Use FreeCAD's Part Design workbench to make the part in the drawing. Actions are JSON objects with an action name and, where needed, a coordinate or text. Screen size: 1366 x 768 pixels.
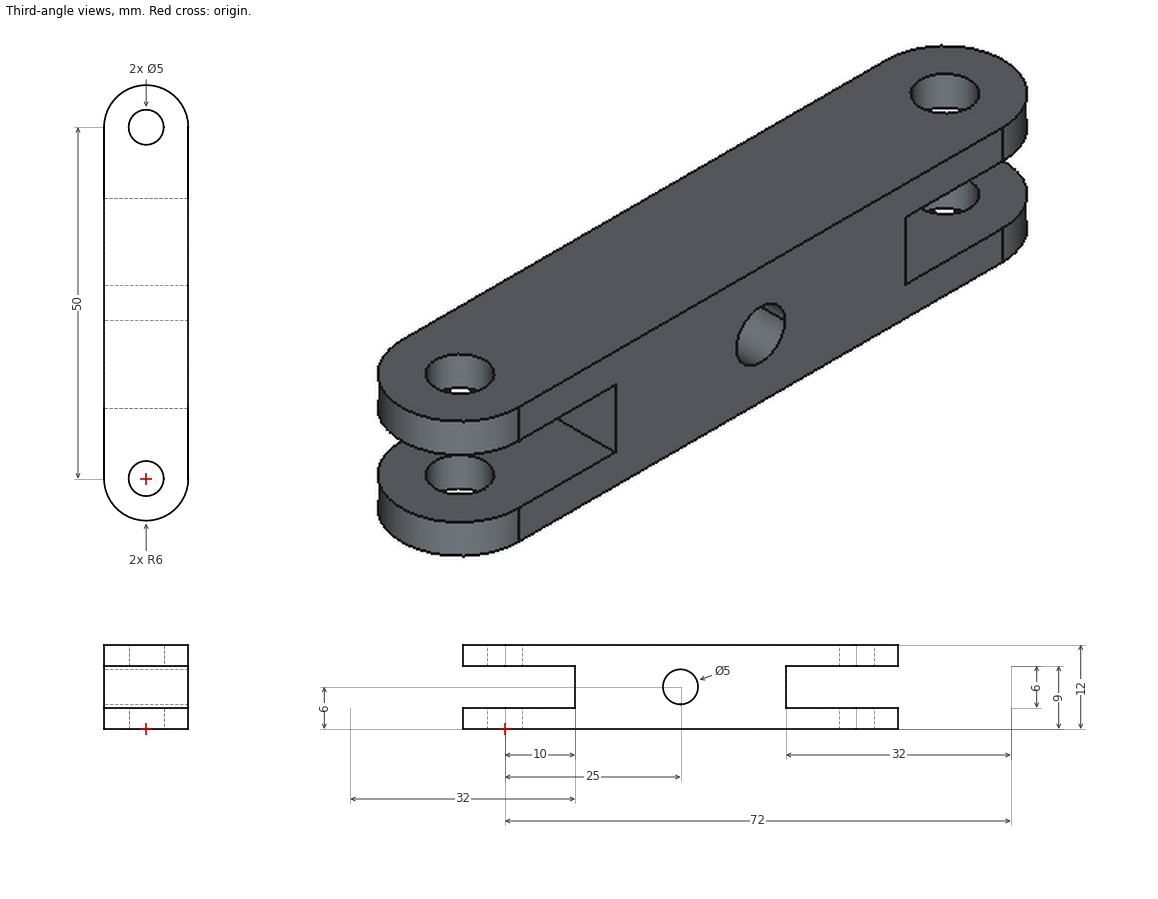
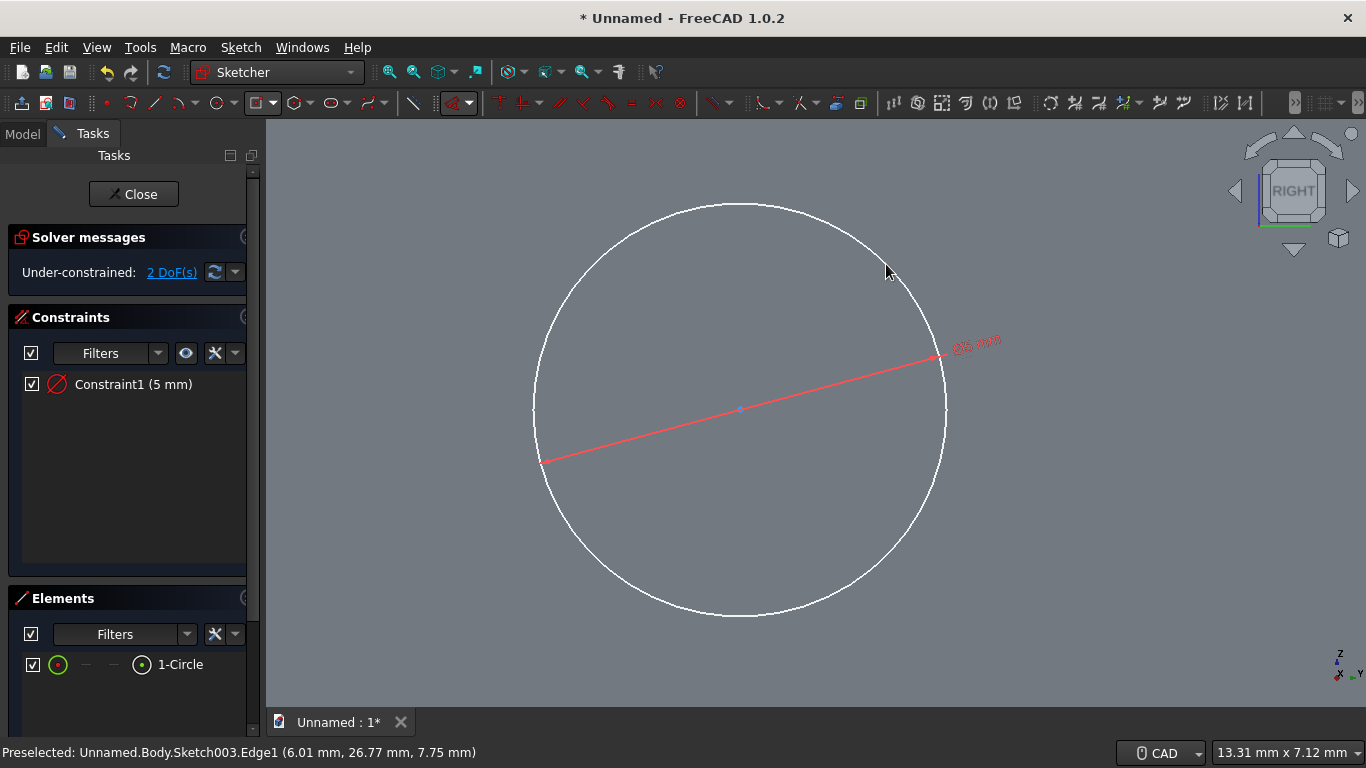
{"action": "left_click", "coordinate": [740, 410]}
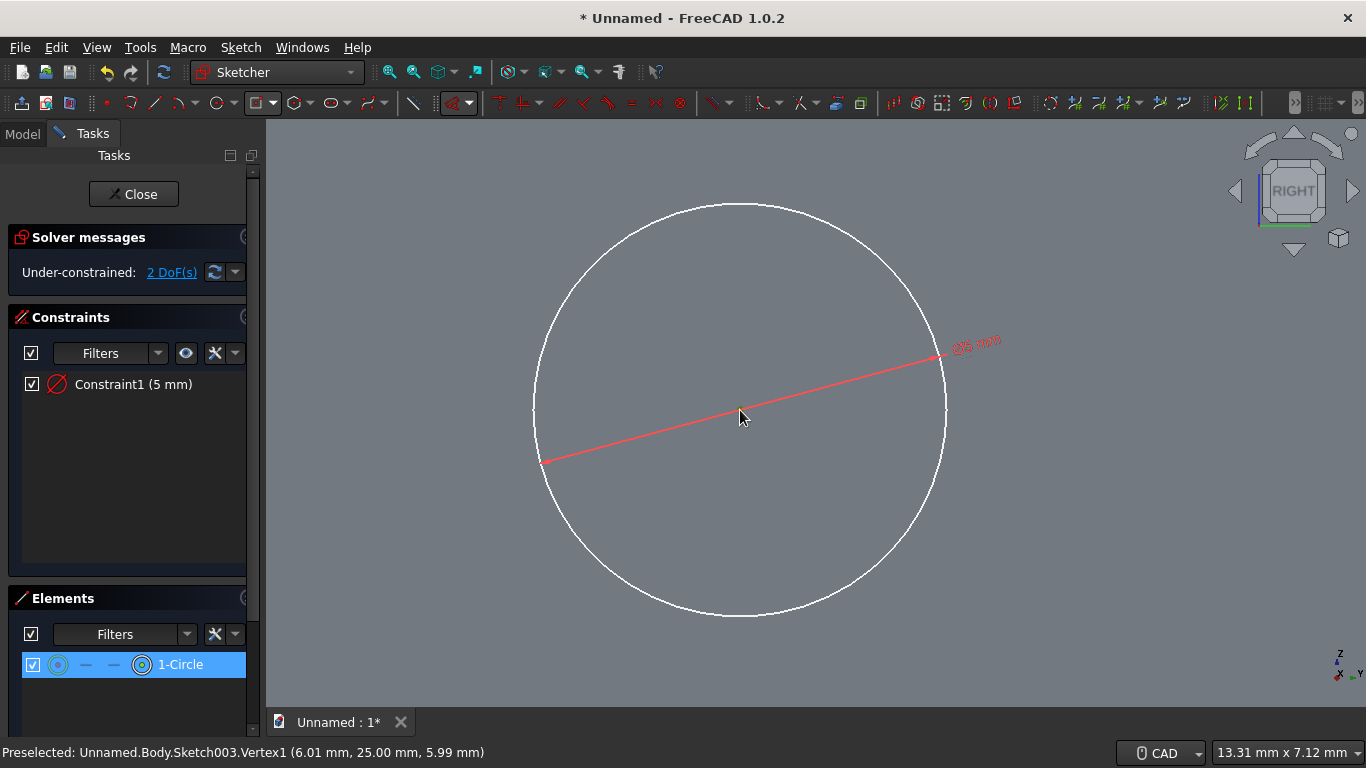
{"action": "left_click", "coordinate": [472, 104]}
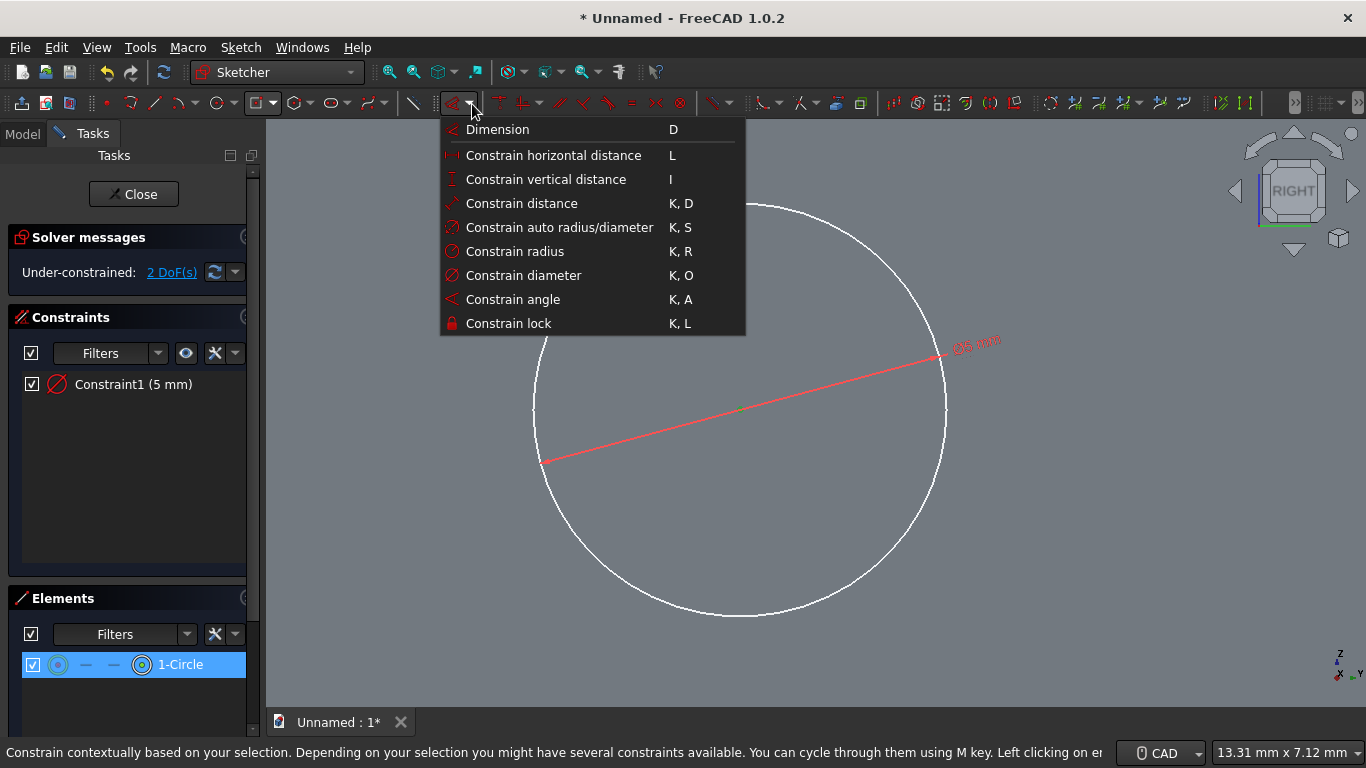
{"action": "left_click", "coordinate": [593, 179]}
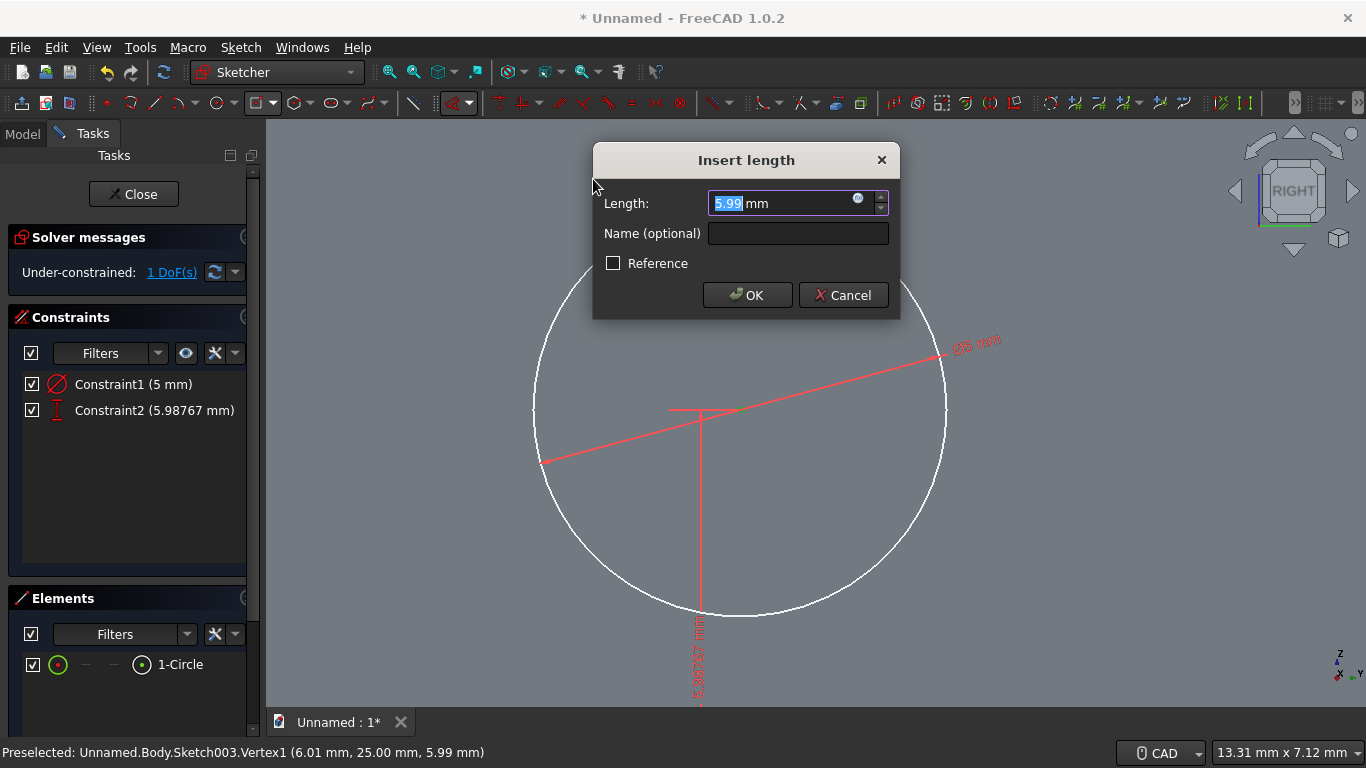
{"action": "type", "text": "6"}
{"action": "key", "text": "Return"}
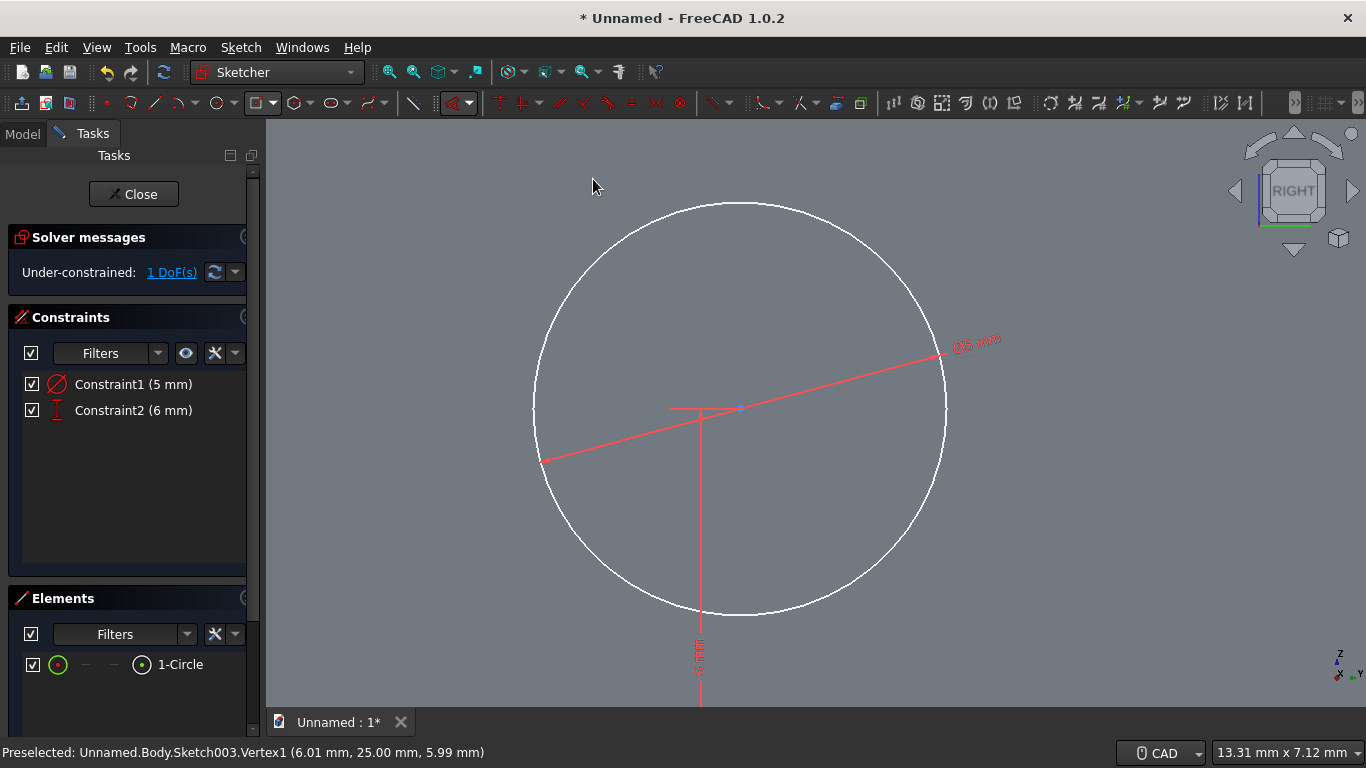
{"action": "left_click", "coordinate": [740, 409]}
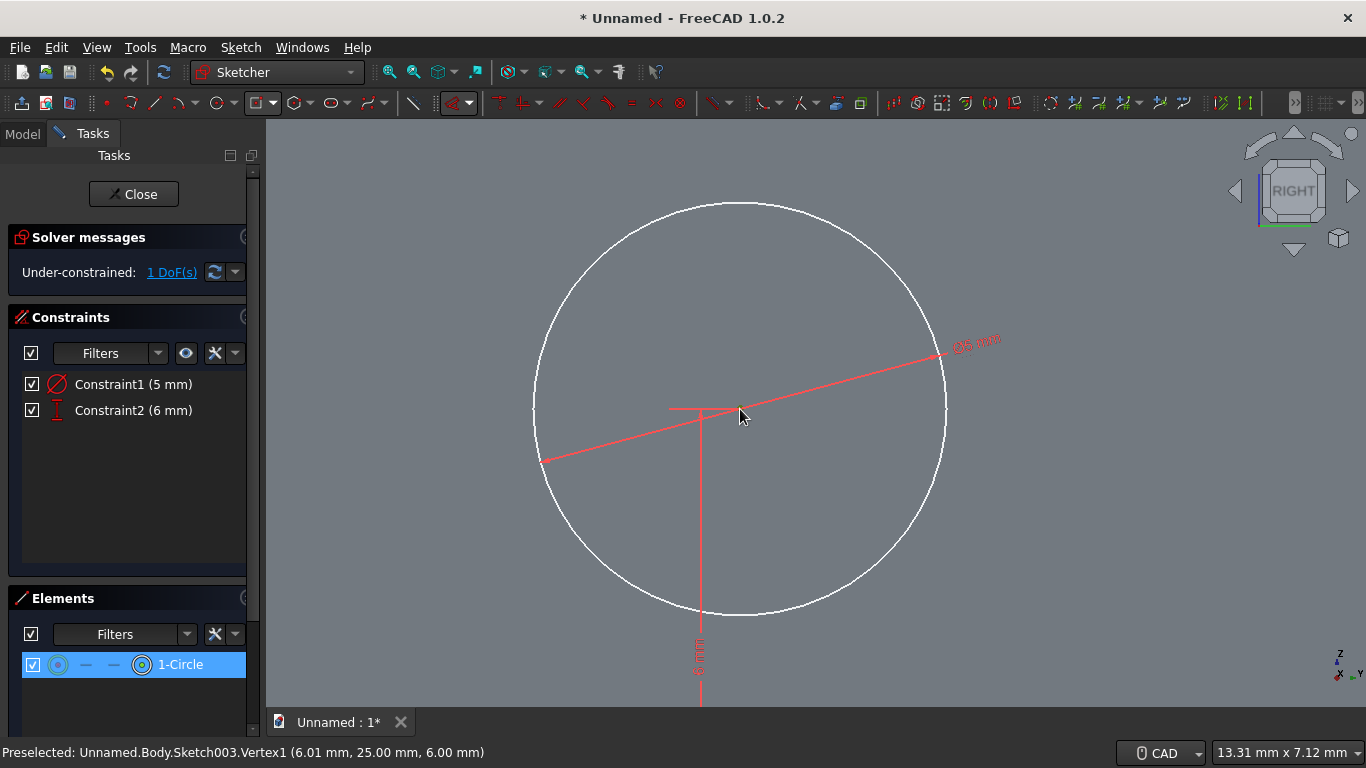
{"action": "left_click", "coordinate": [472, 104]}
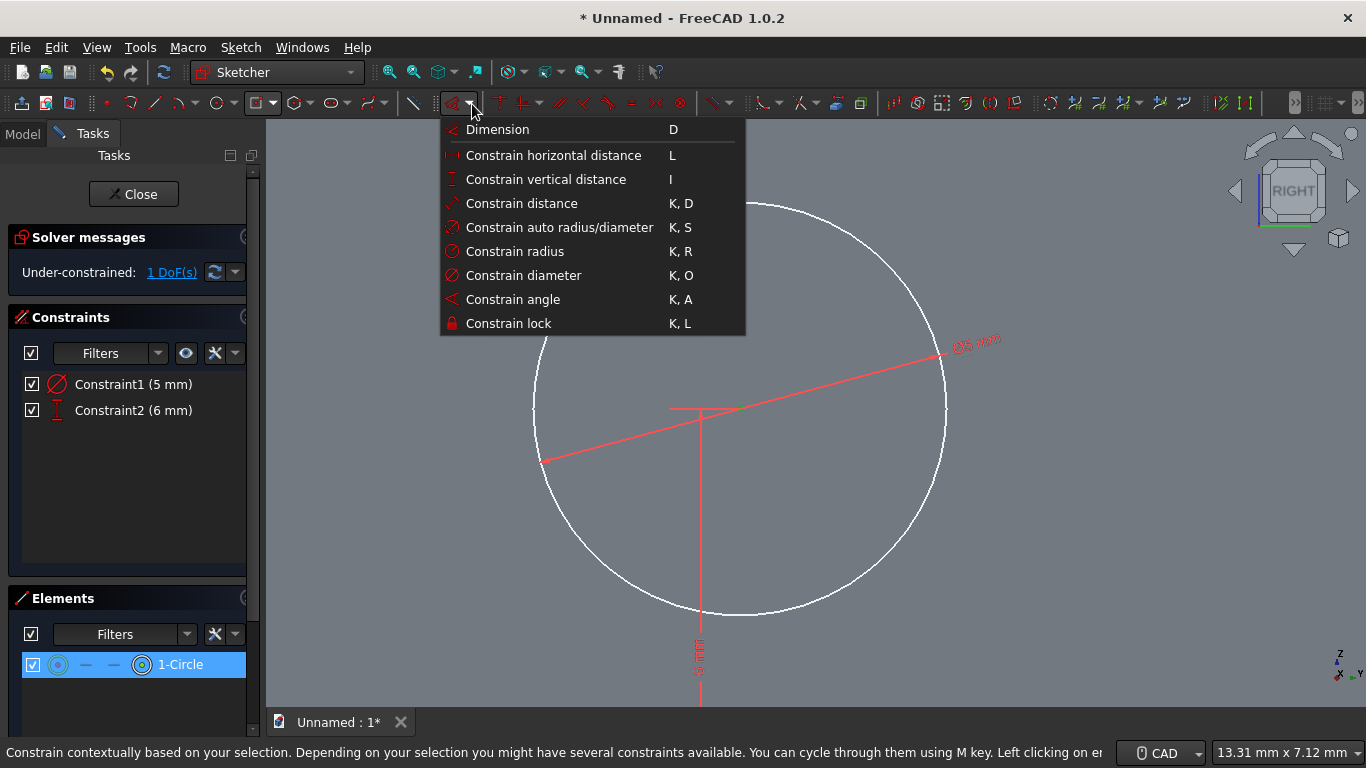
{"action": "left_click", "coordinate": [593, 155]}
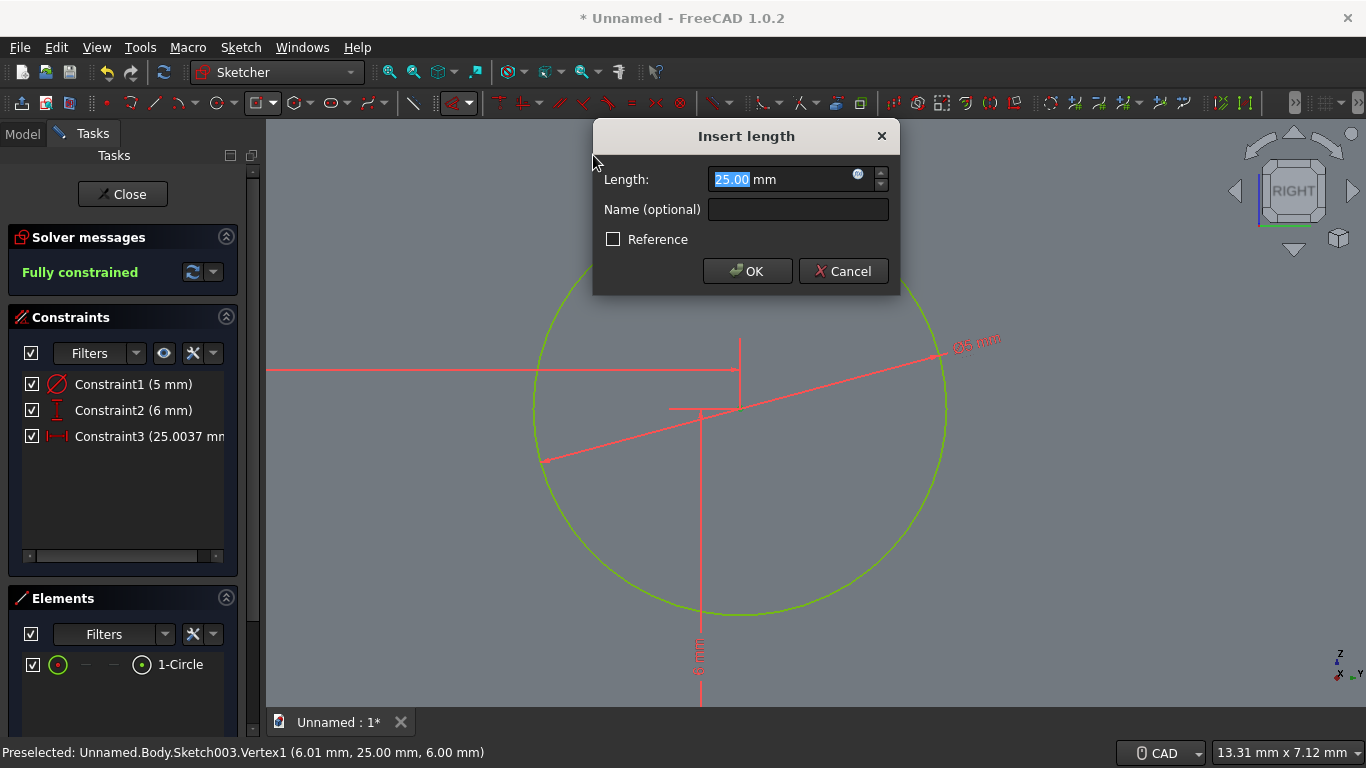
{"action": "type", "text": "25"}
{"action": "key", "text": "Return"}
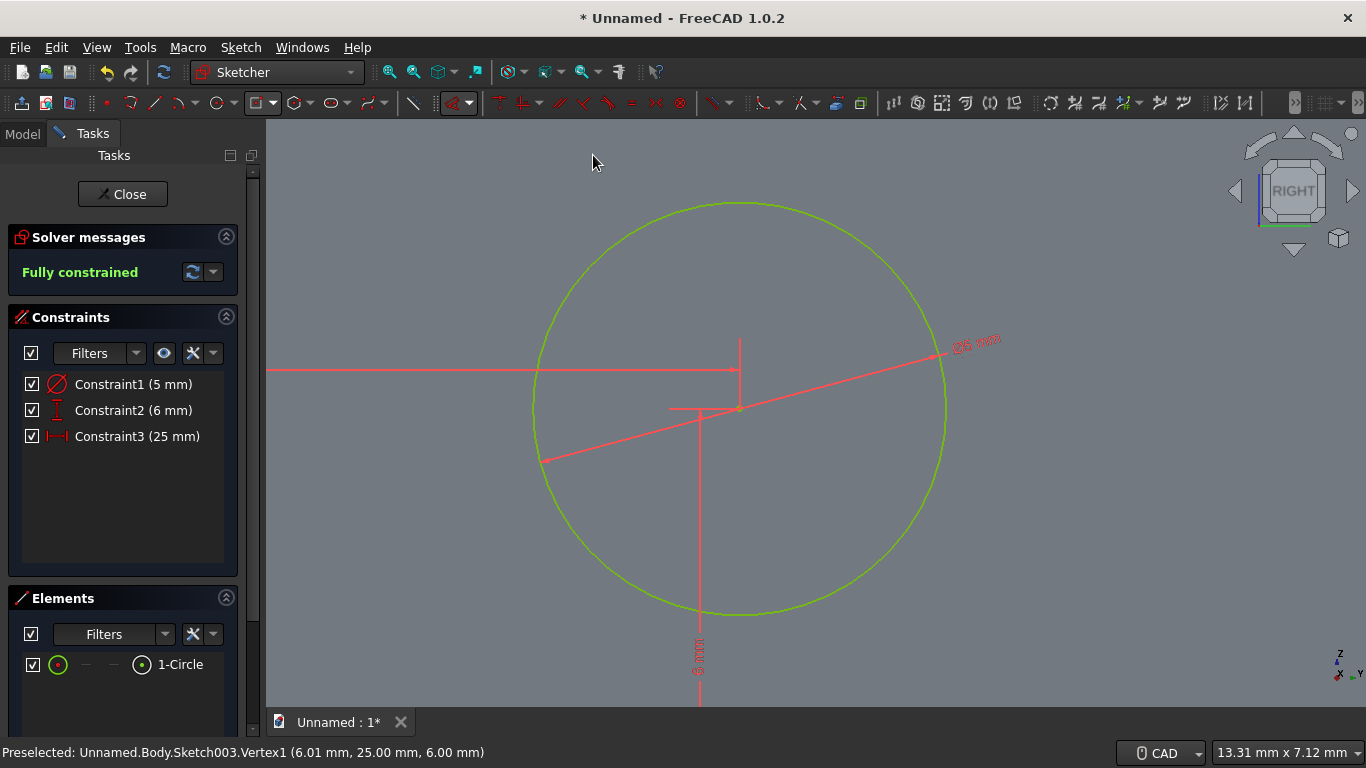
{"action": "left_click", "coordinate": [123, 194]}